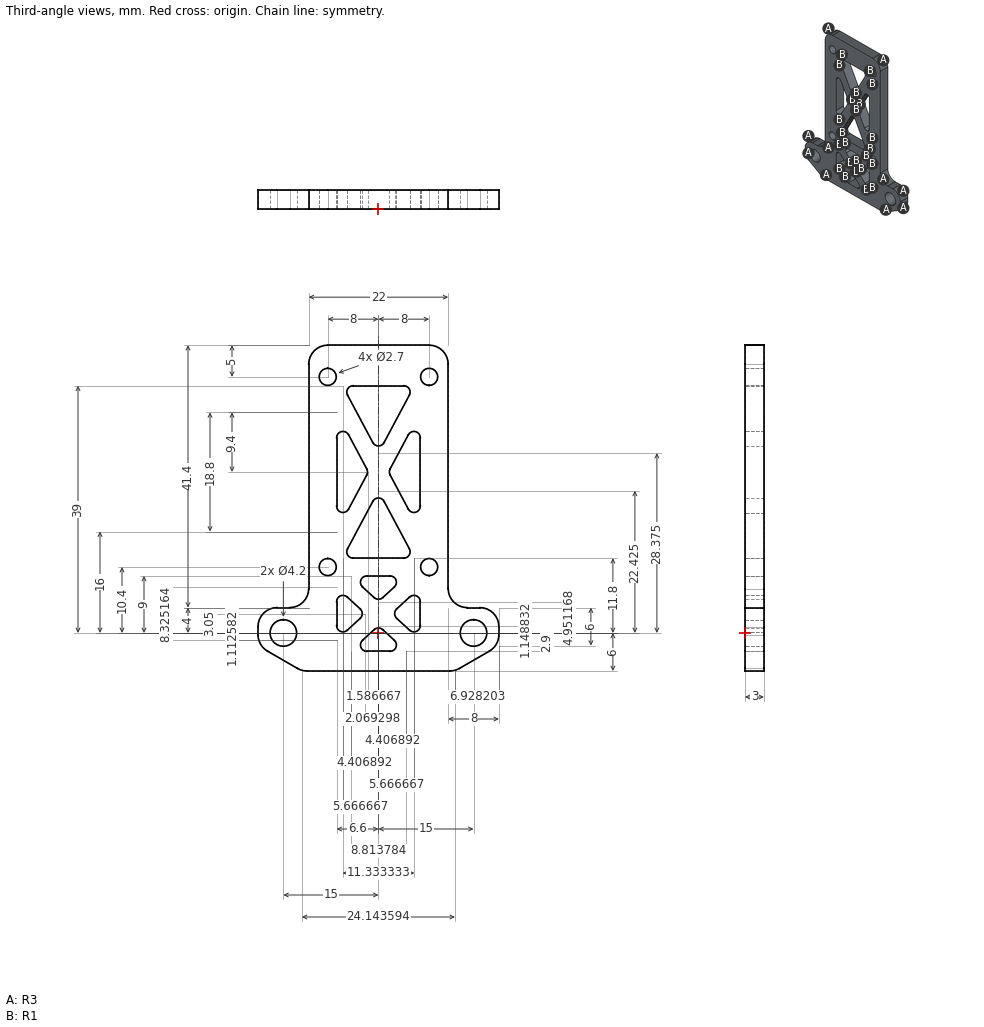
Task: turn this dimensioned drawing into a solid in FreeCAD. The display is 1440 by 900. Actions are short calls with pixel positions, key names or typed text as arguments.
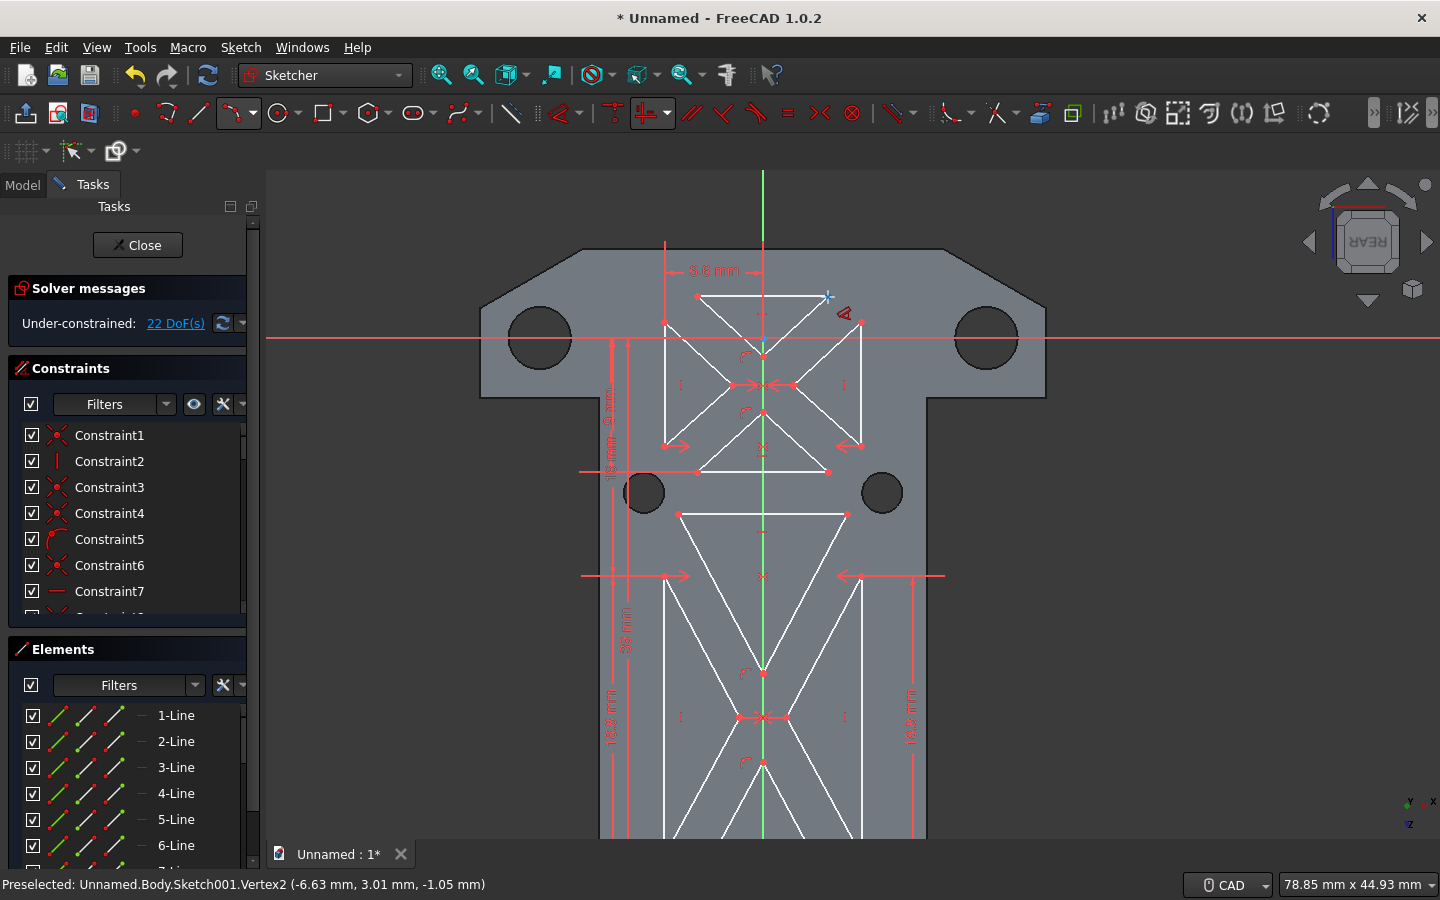
click(828, 296)
click(862, 308)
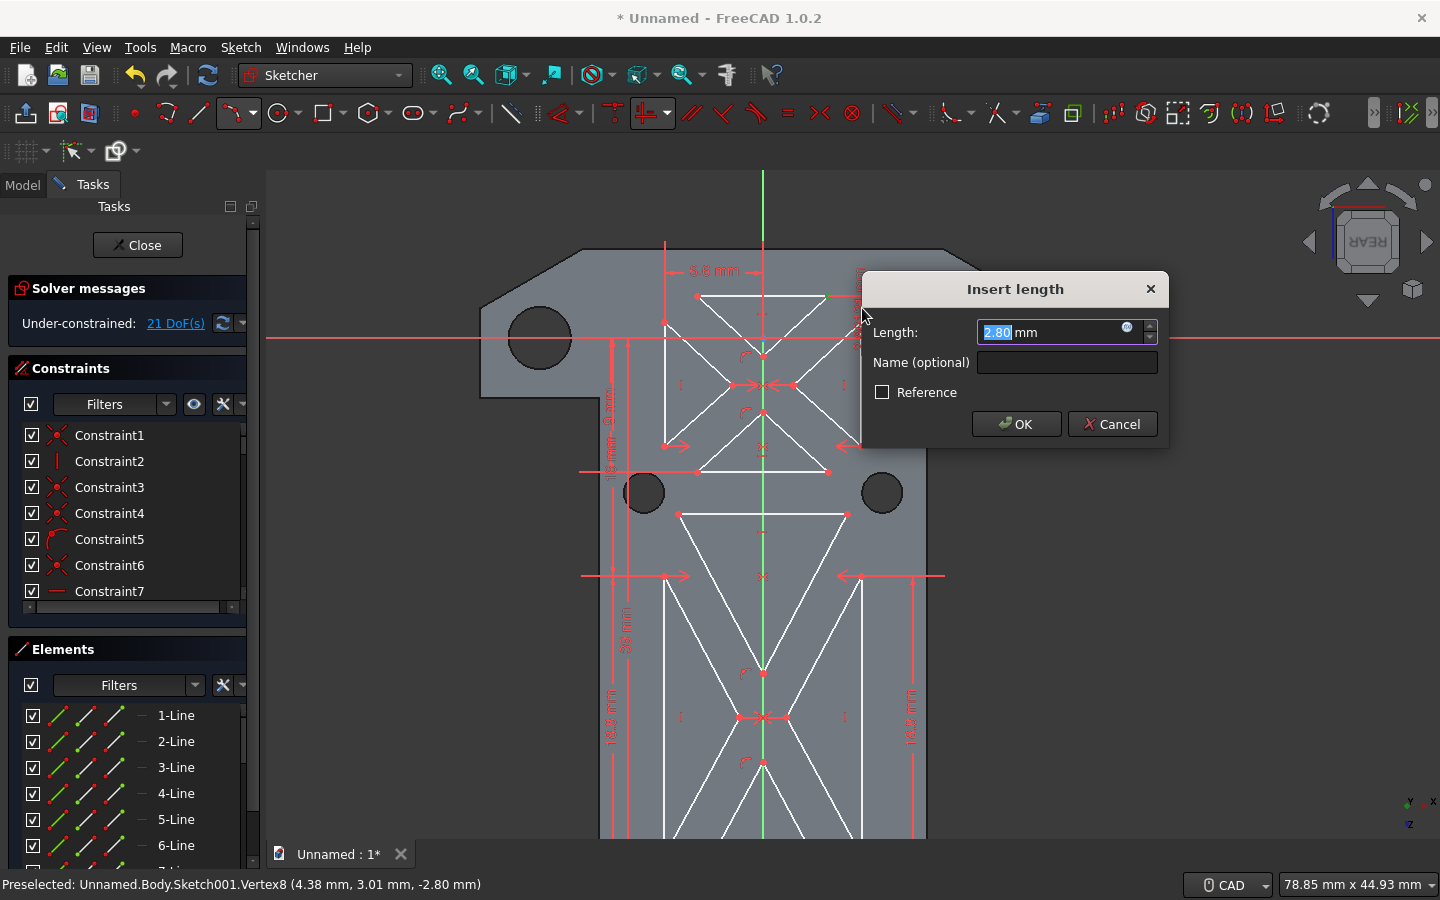
text(2.9)
key(Return)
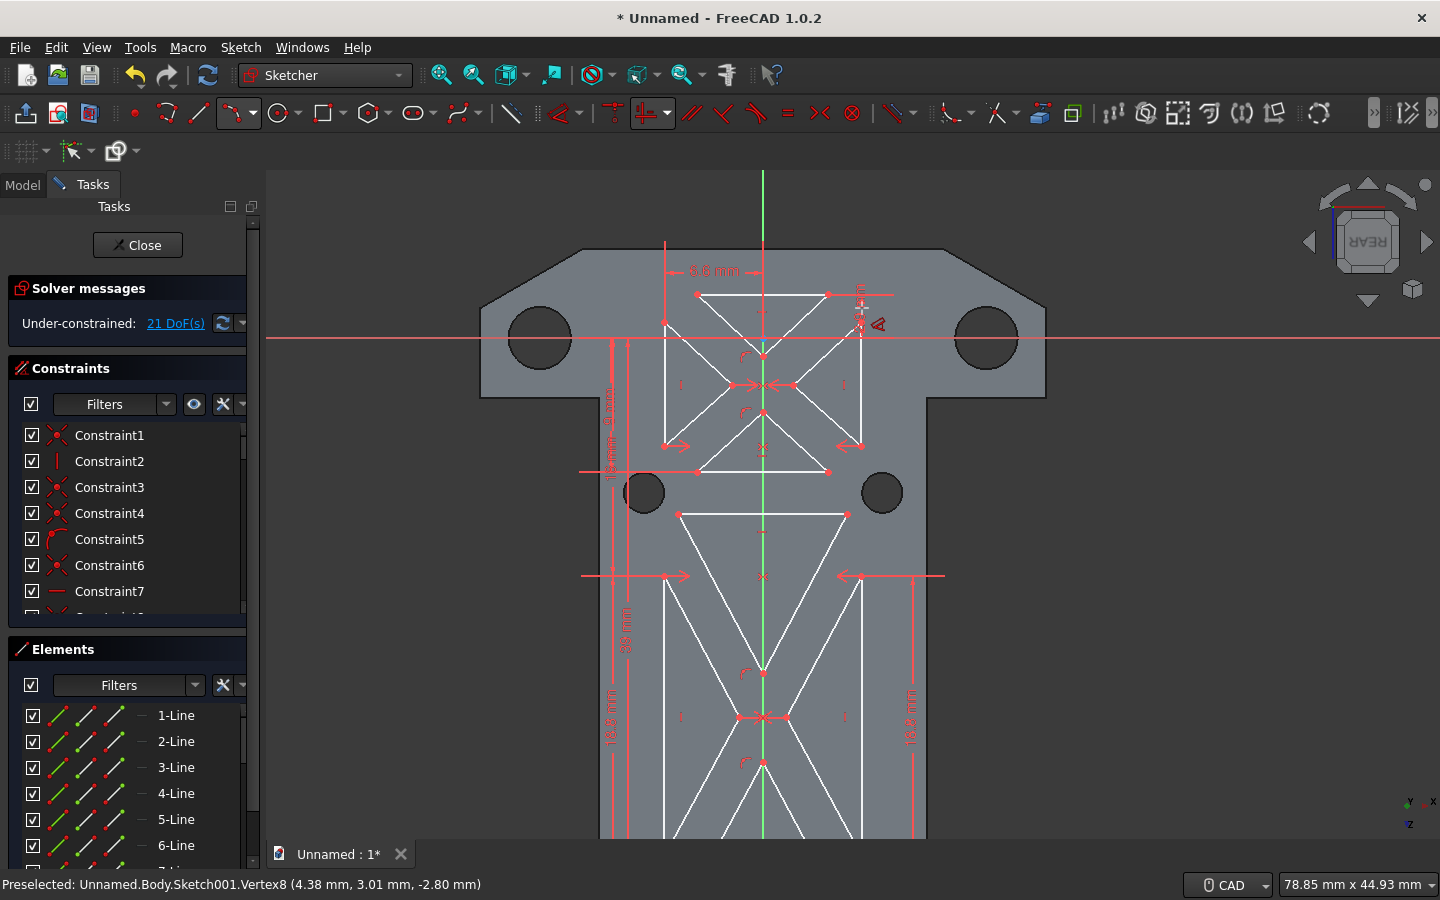
click(664, 576)
click(679, 304)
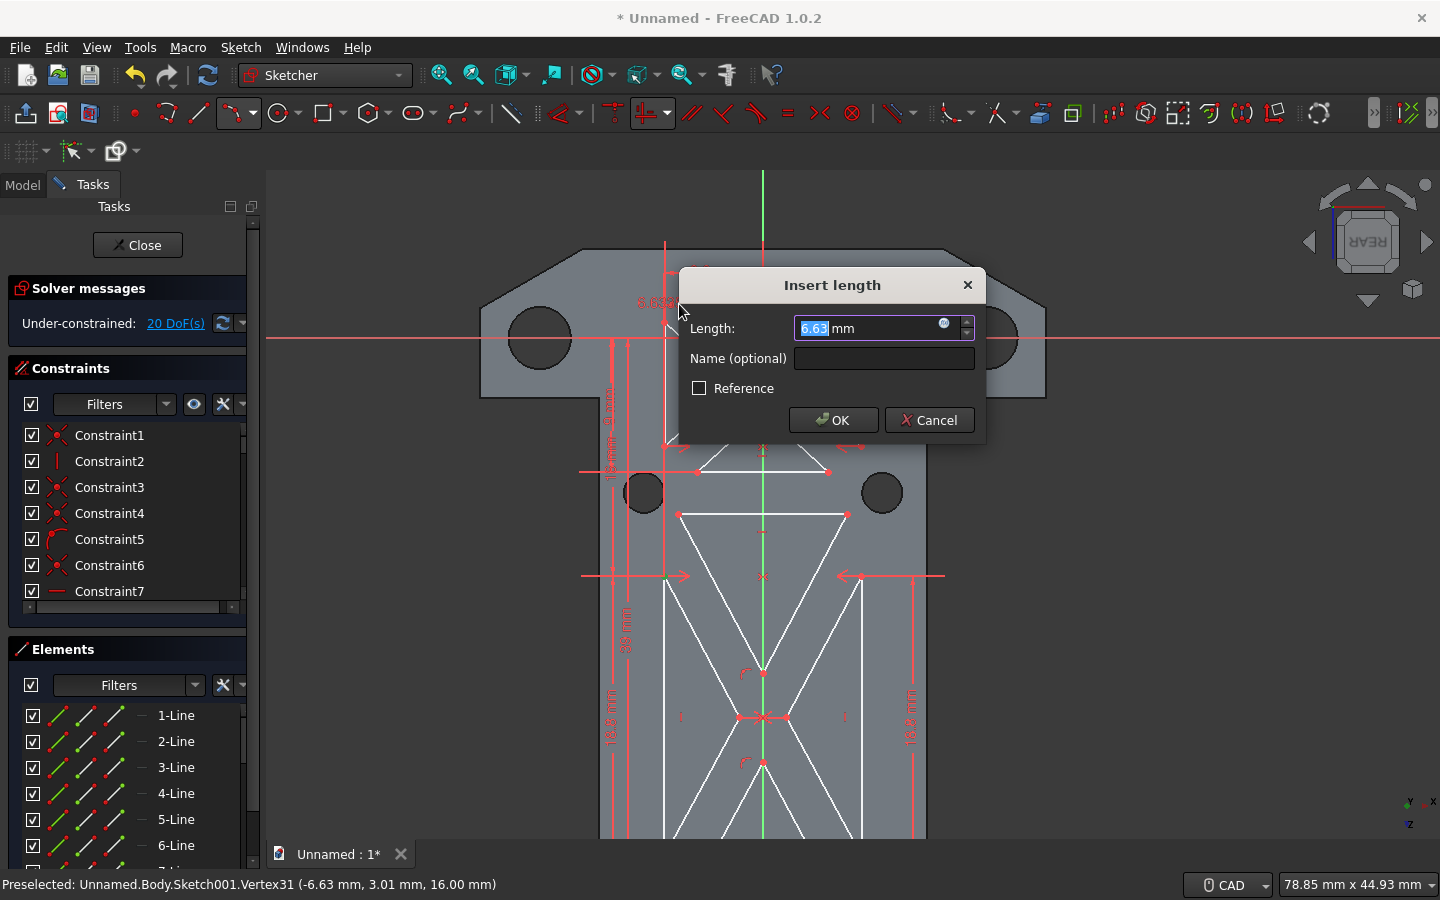
text(6.6)
key(Return)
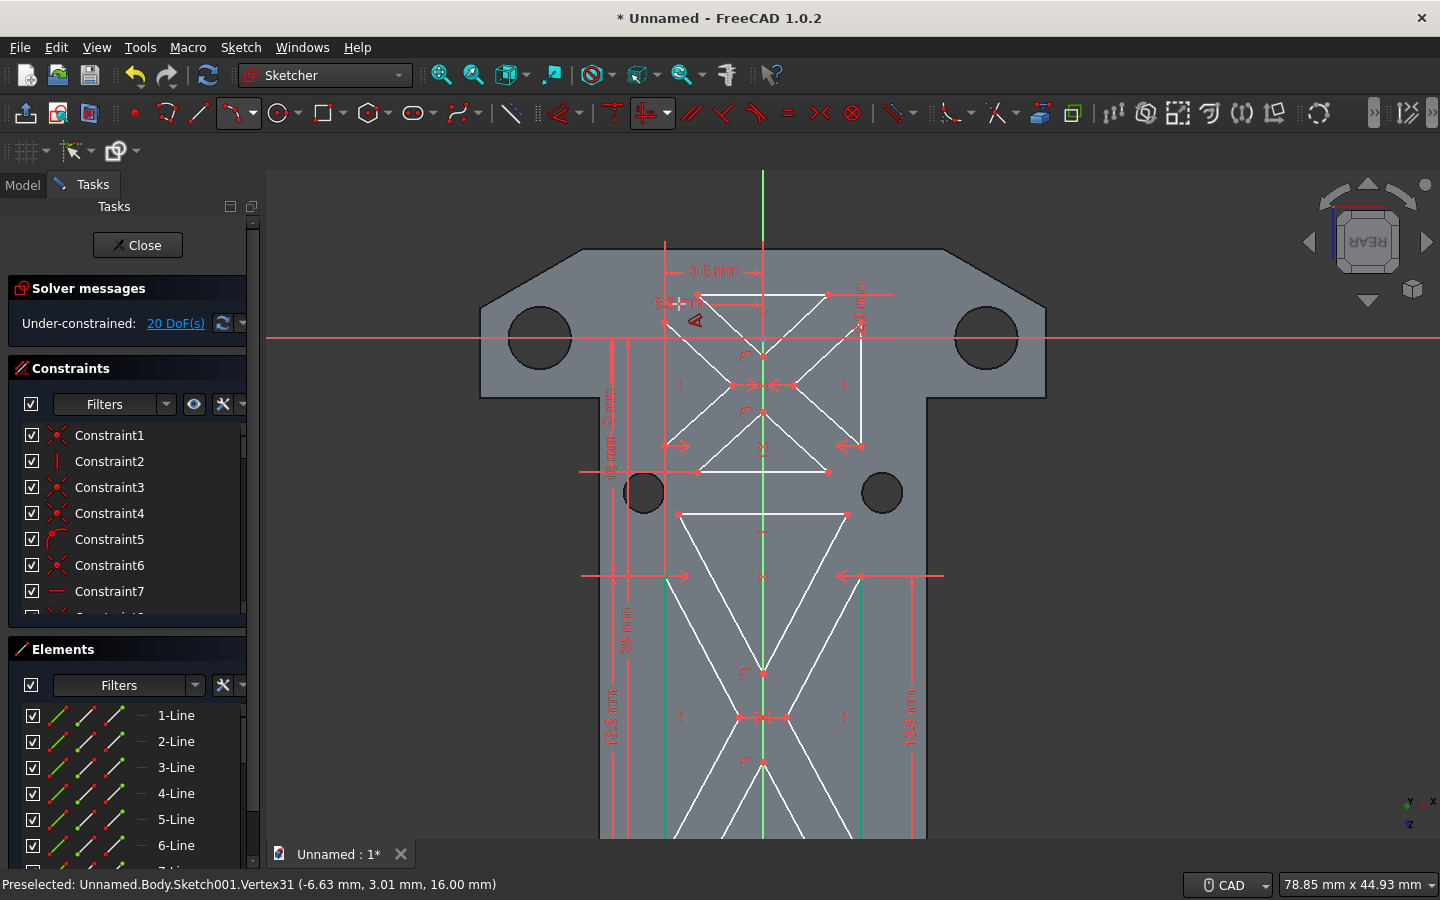
click(717, 759)
click(631, 764)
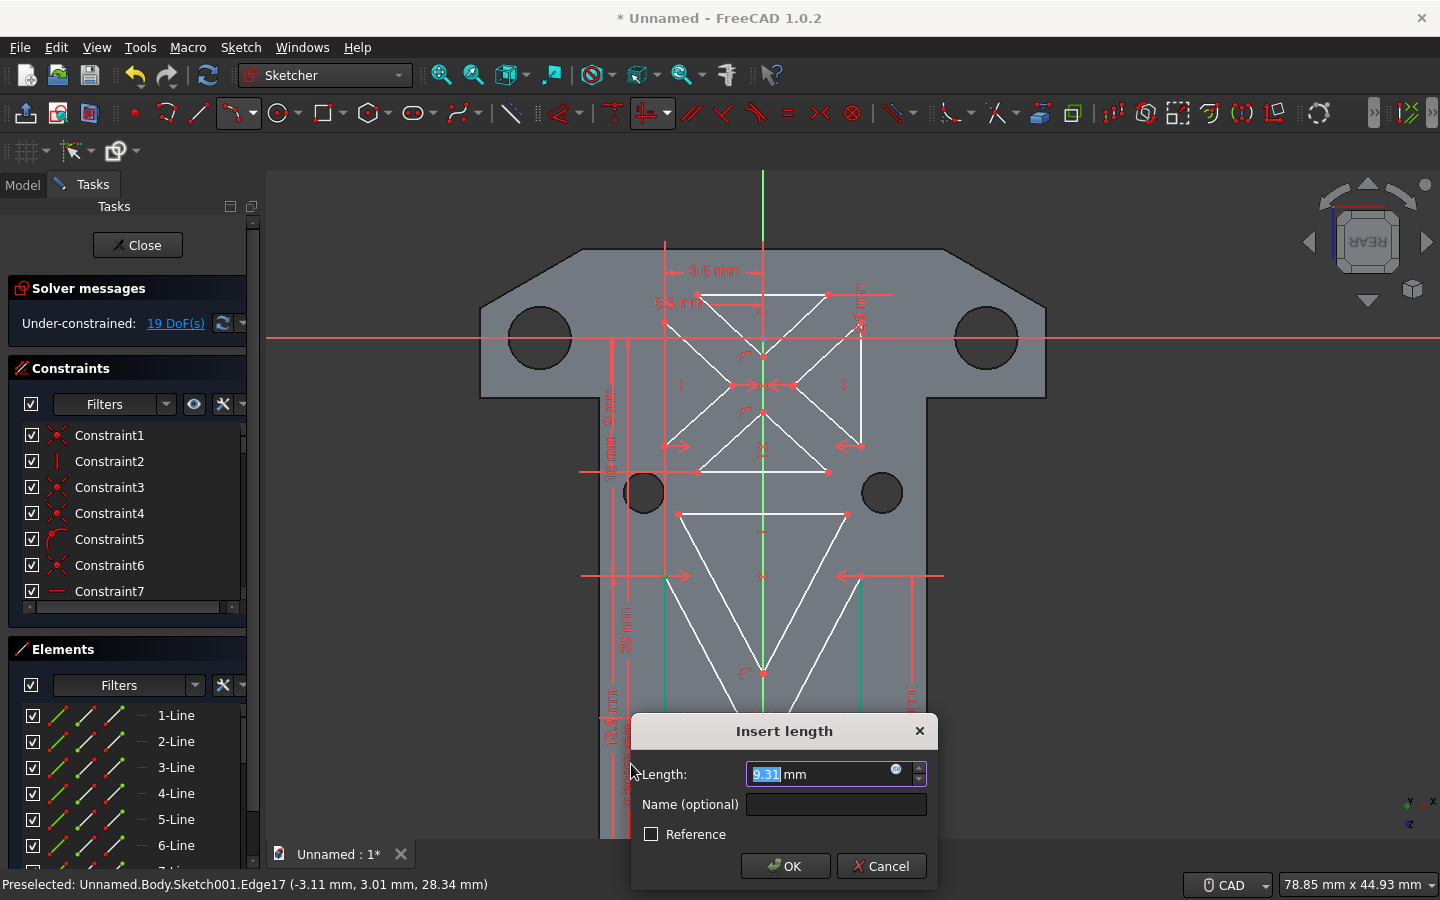
text(9.4)
key(Return)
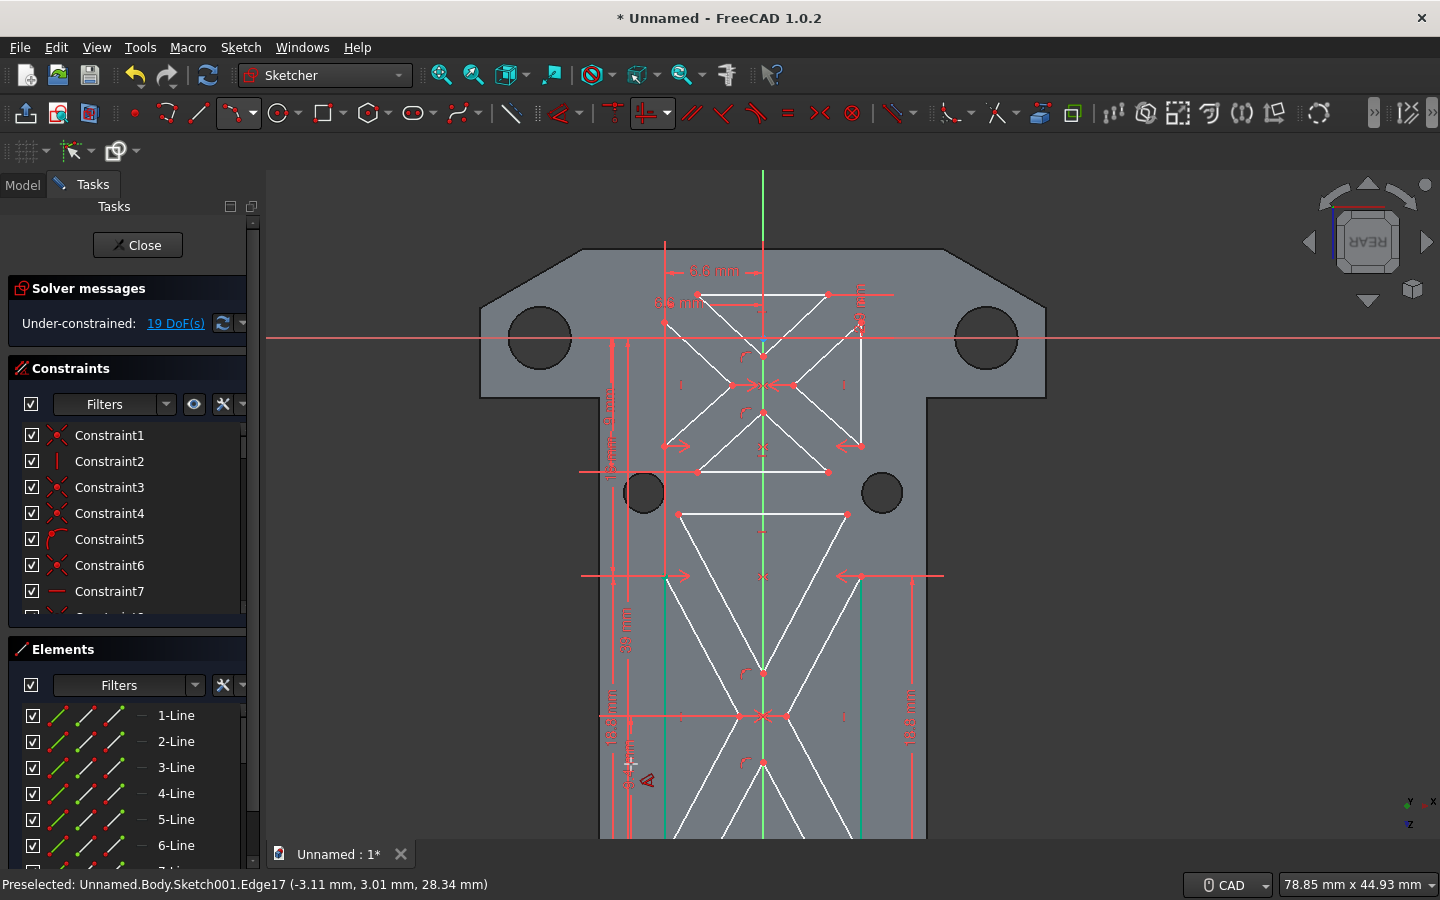
click(733, 385)
click(699, 373)